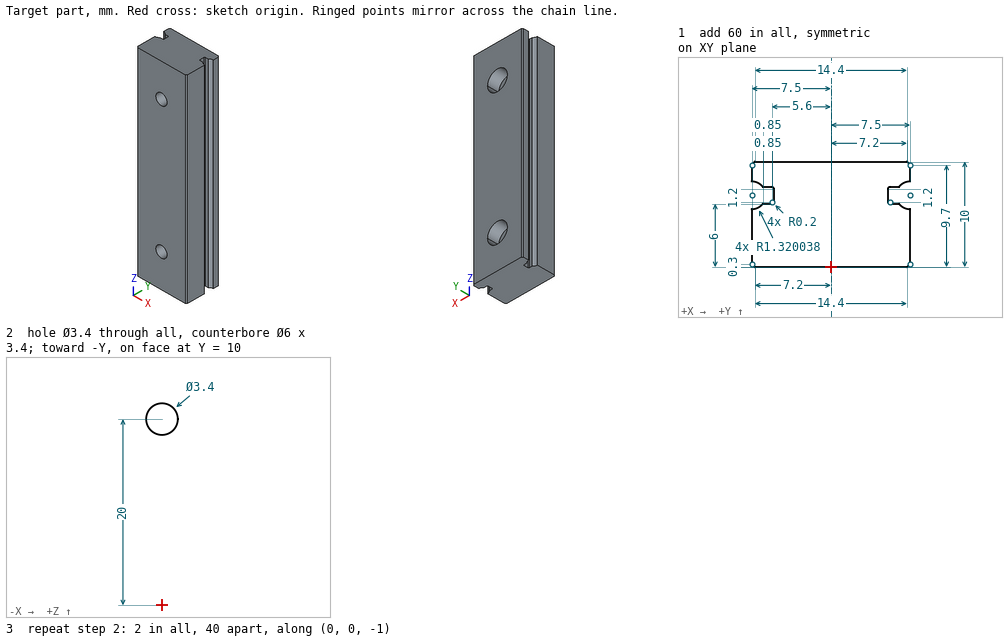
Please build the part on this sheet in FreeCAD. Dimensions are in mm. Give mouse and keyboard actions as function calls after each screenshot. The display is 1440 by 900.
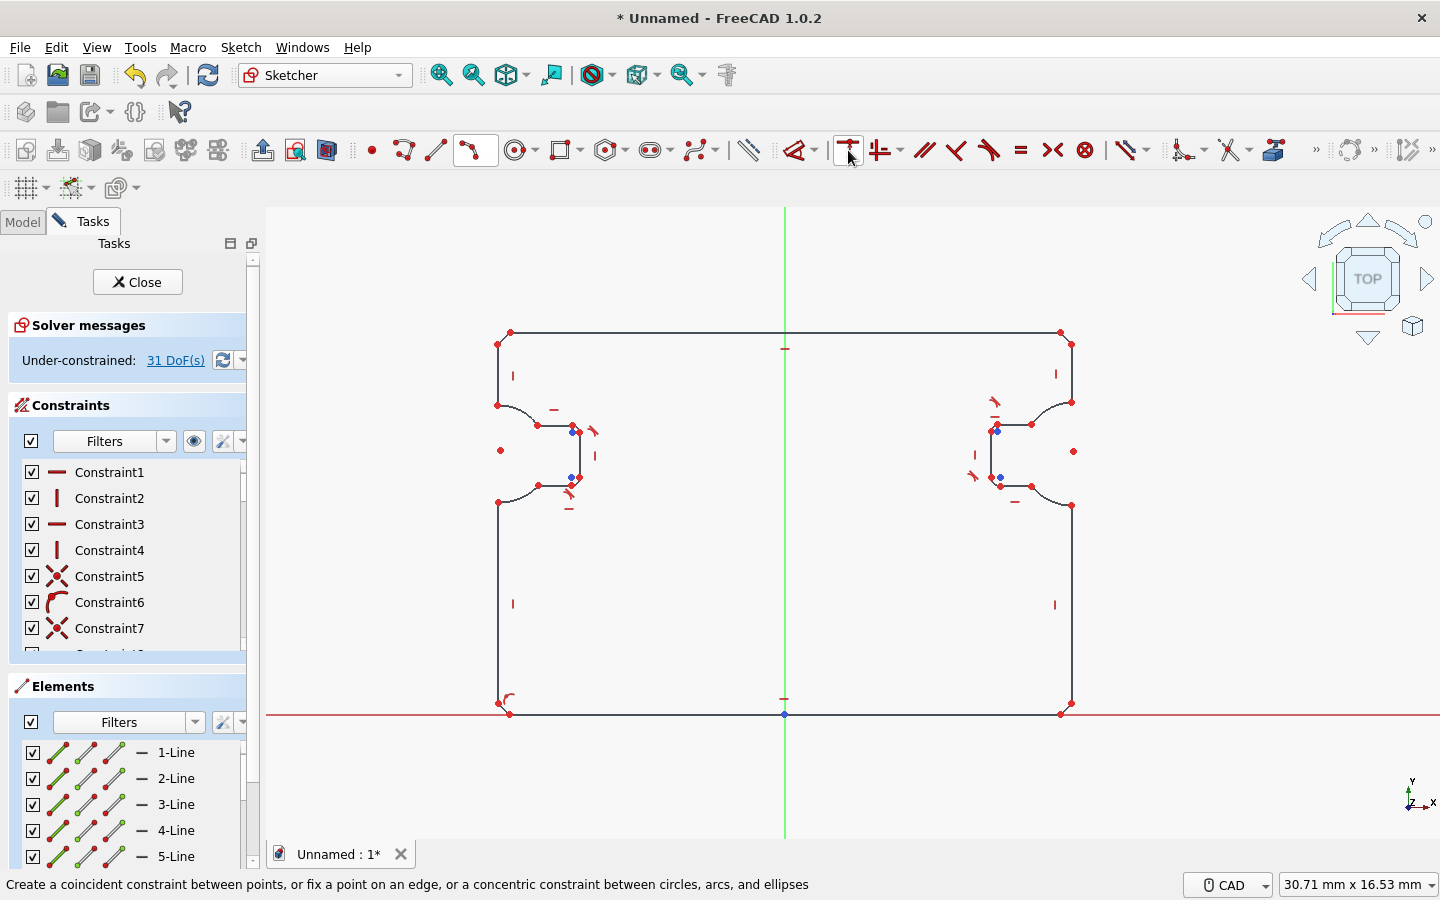
scroll(577, 428, up, 5)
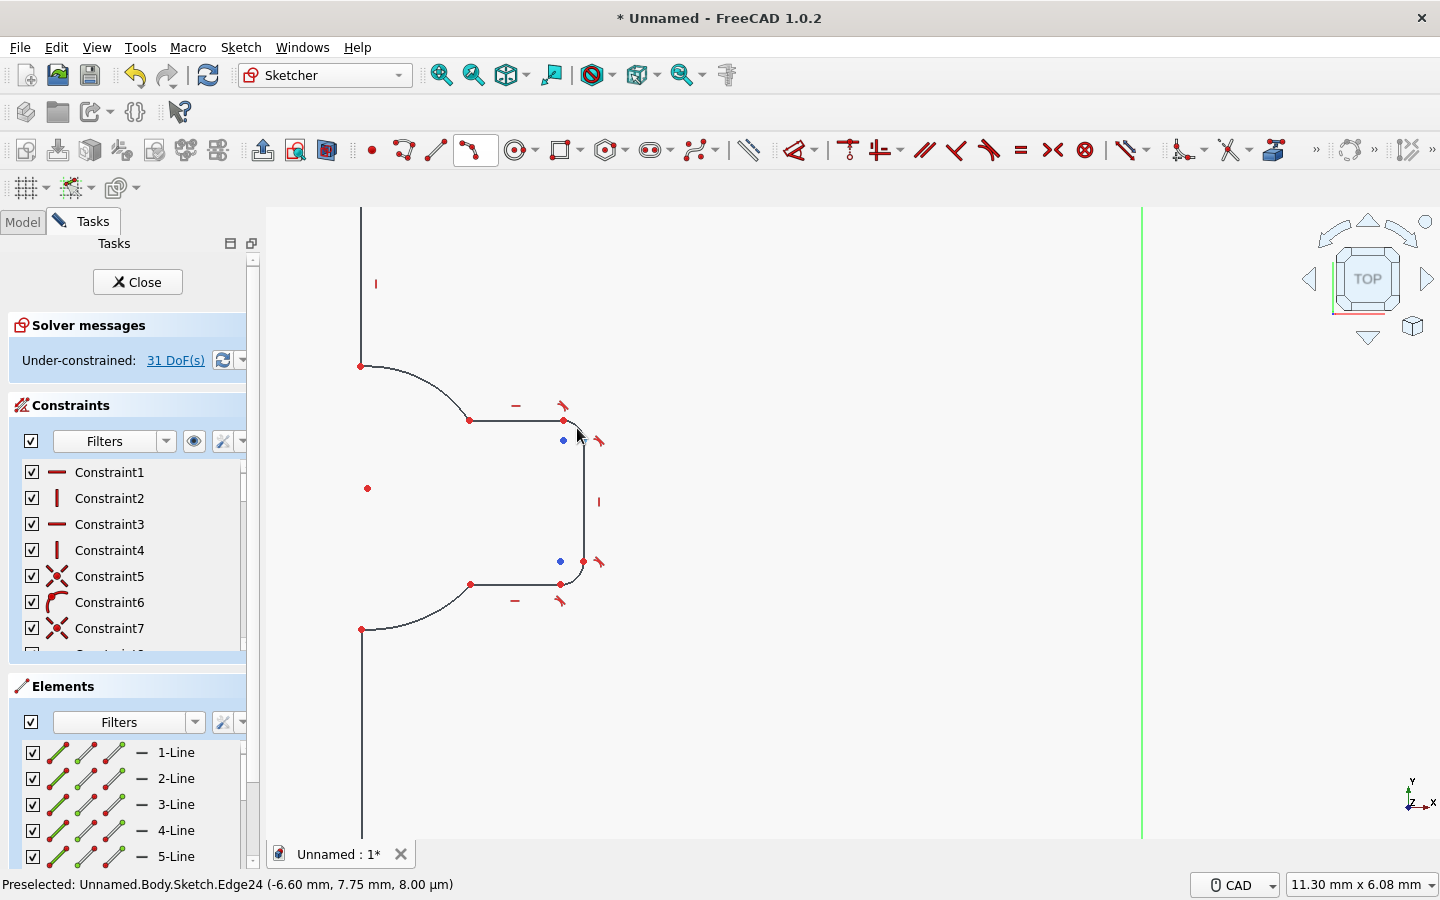
click(578, 427)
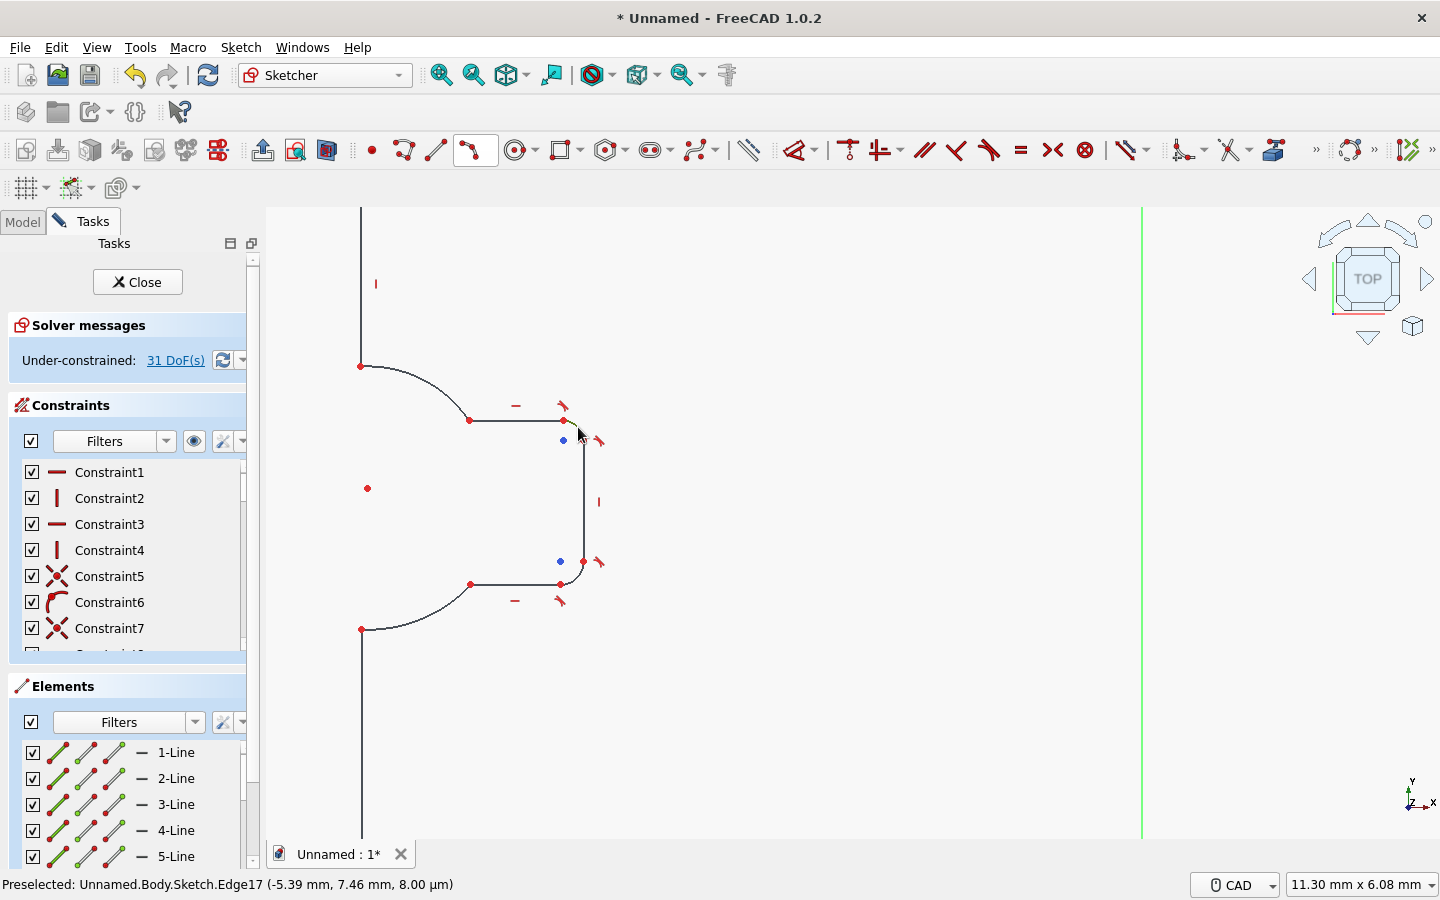
scroll(571, 582, up, 2)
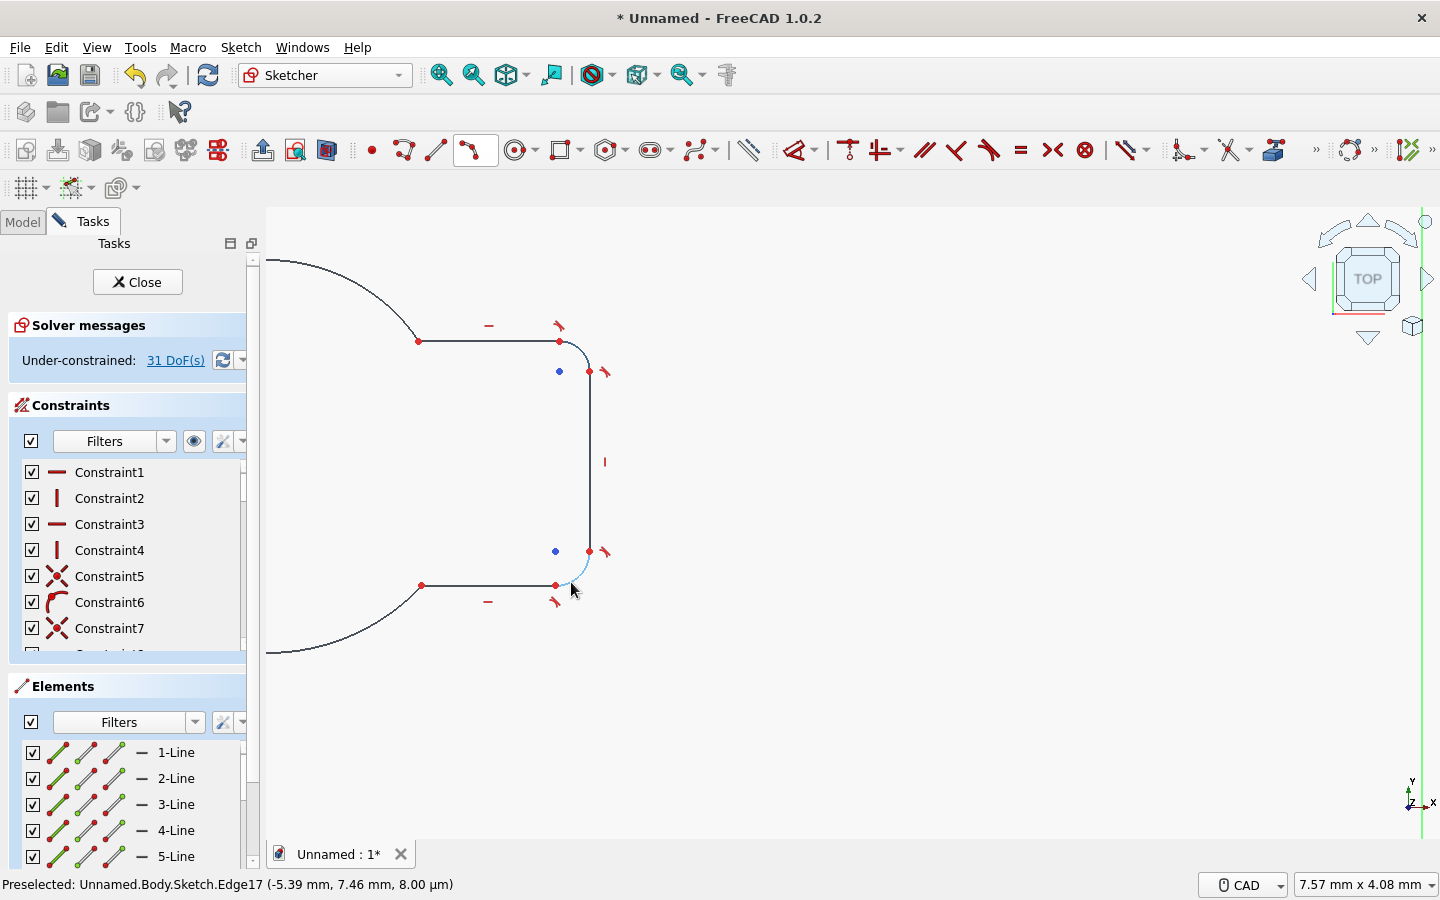
click(571, 582)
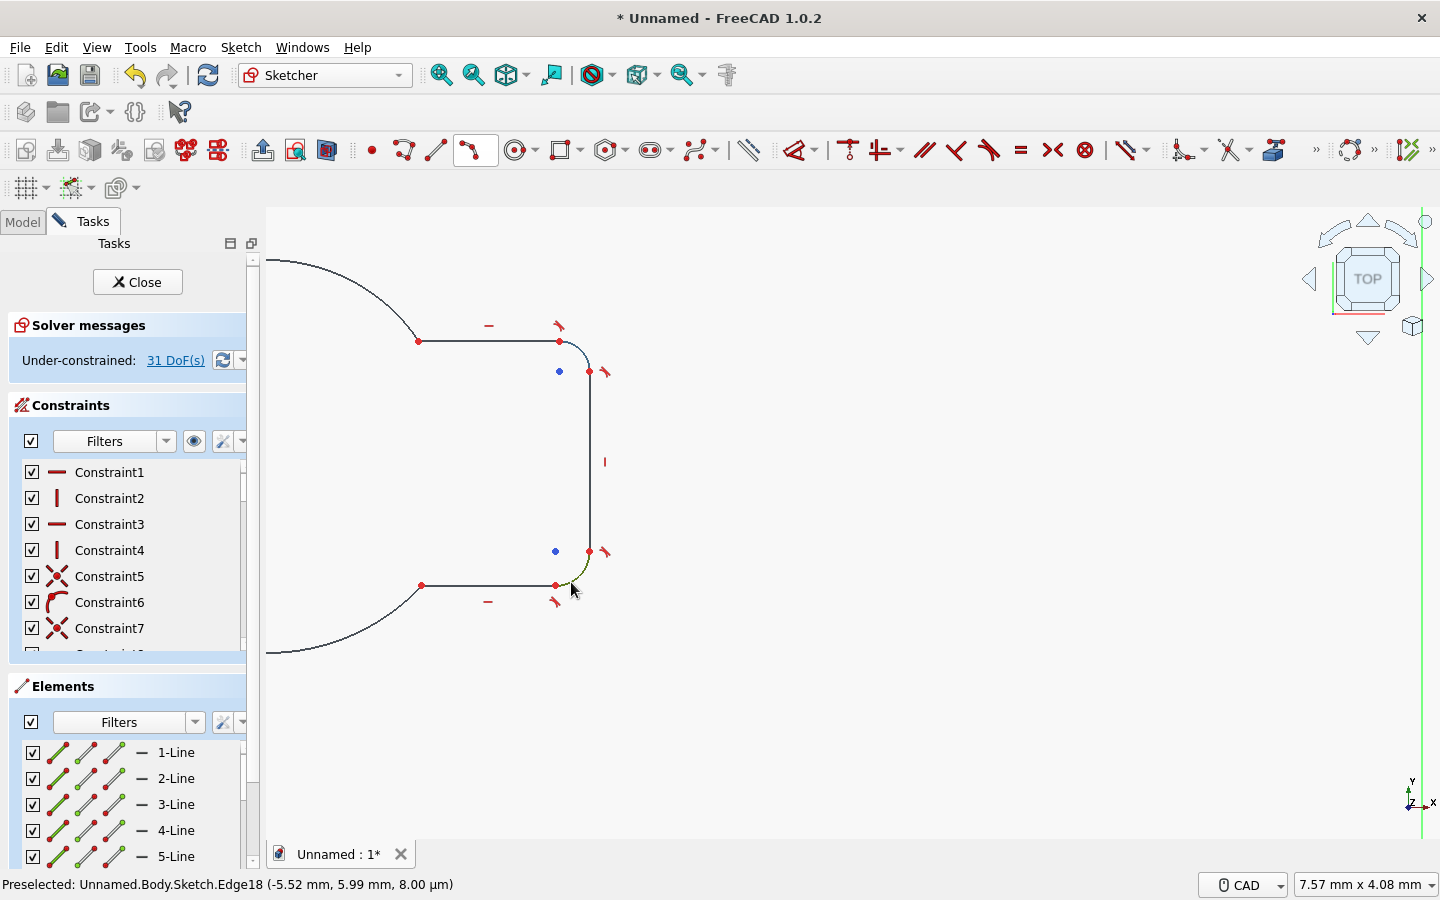
scroll(576, 453, down, 7)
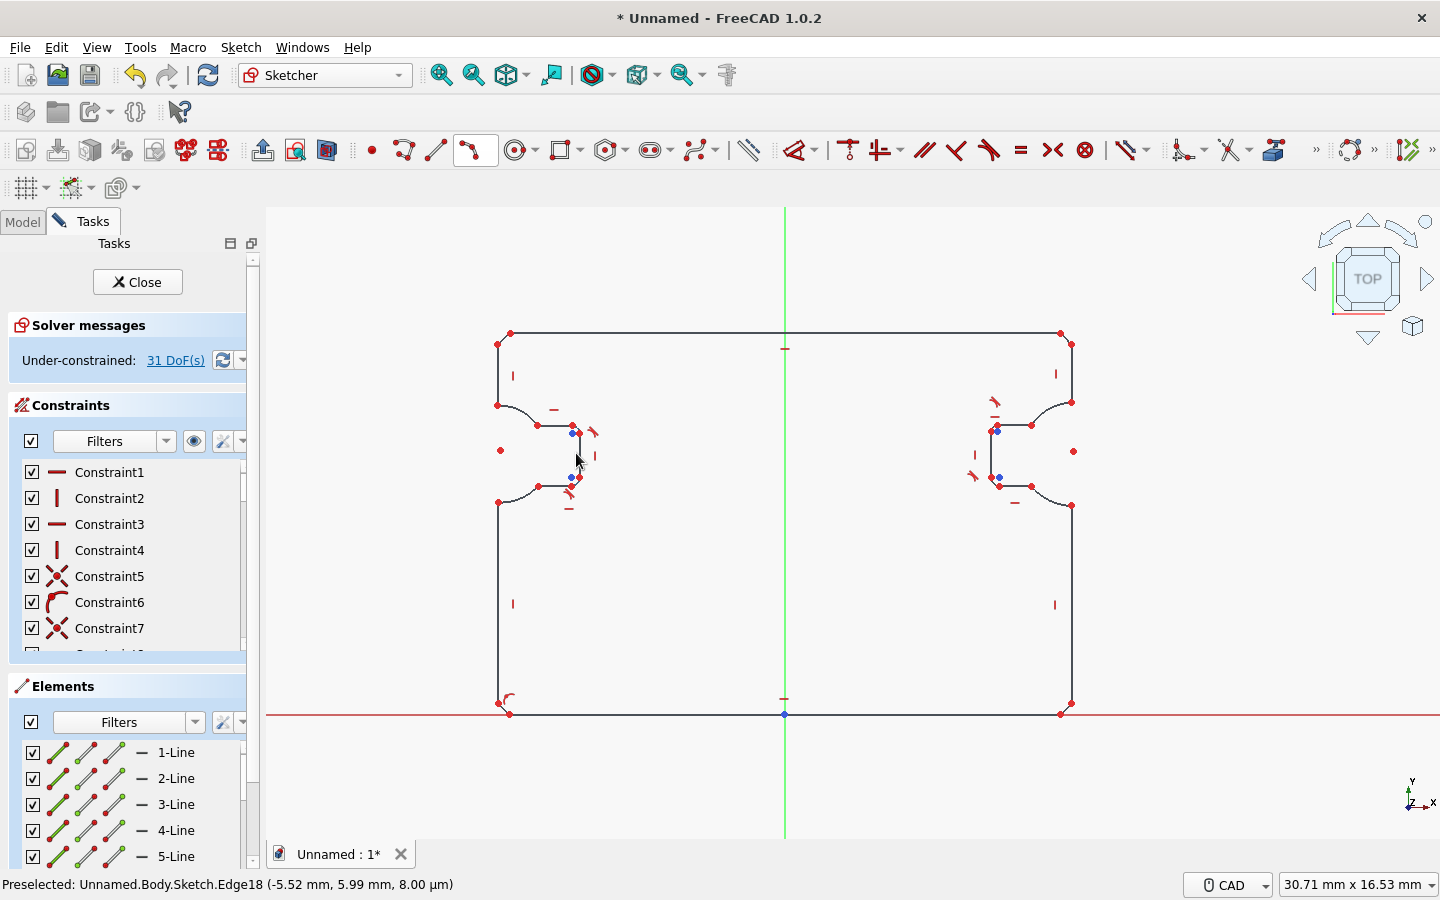
scroll(992, 481, up, 7)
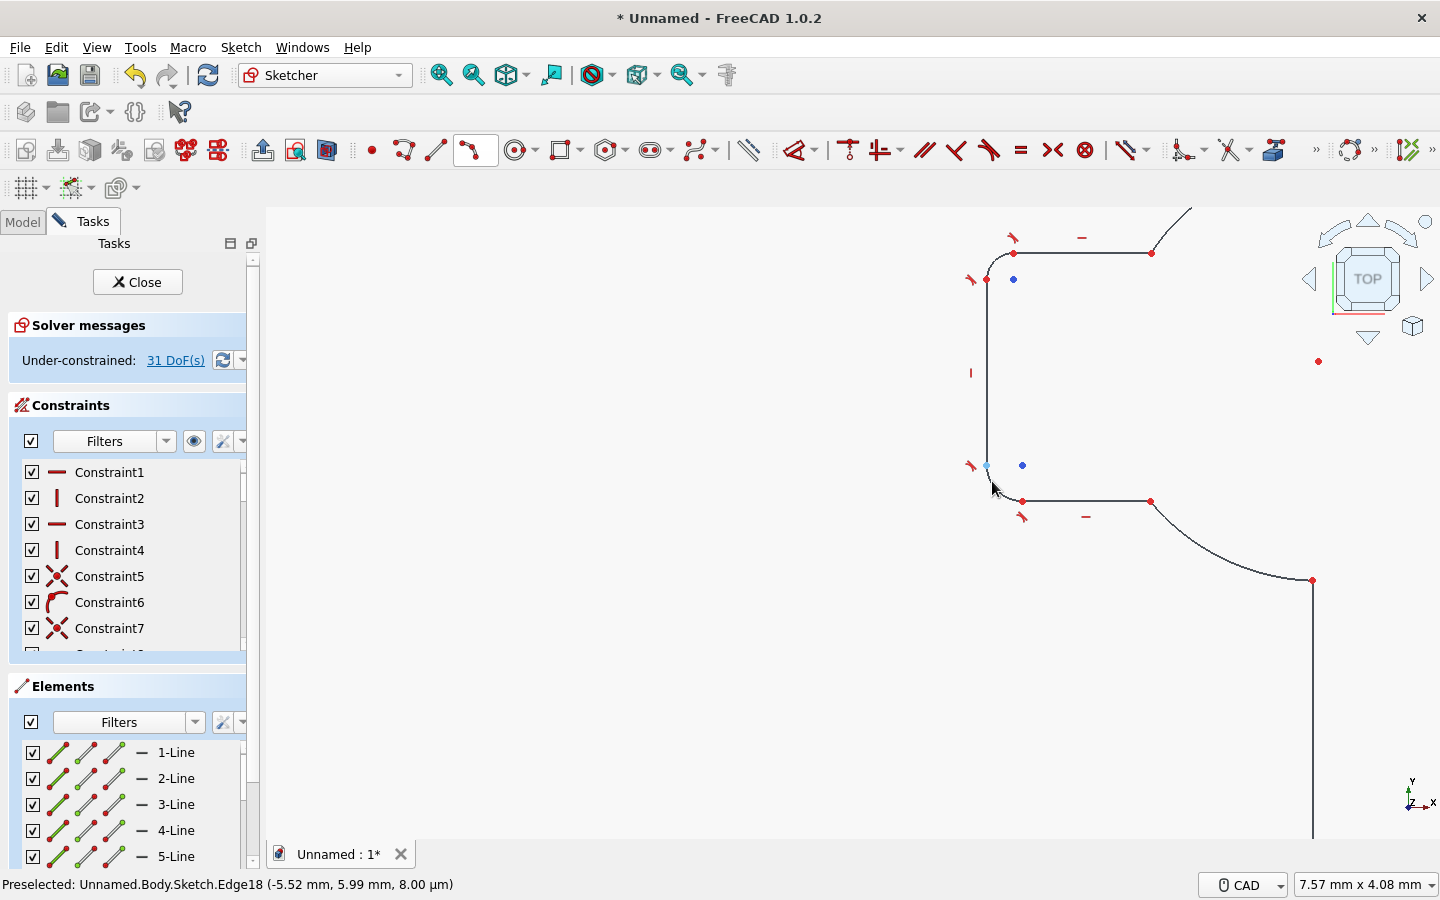
click(991, 482)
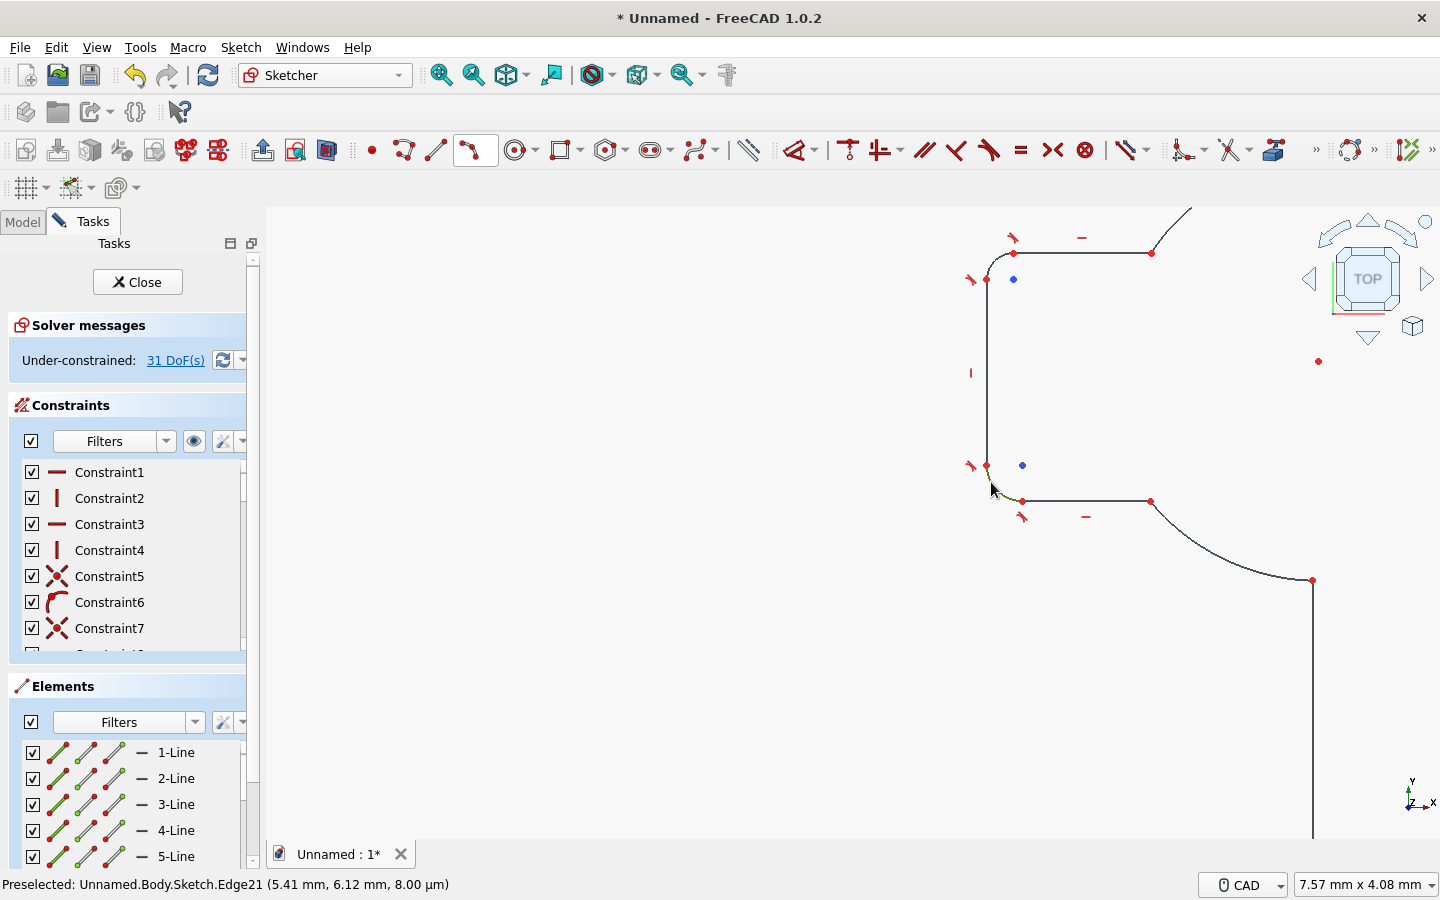
click(1002, 256)